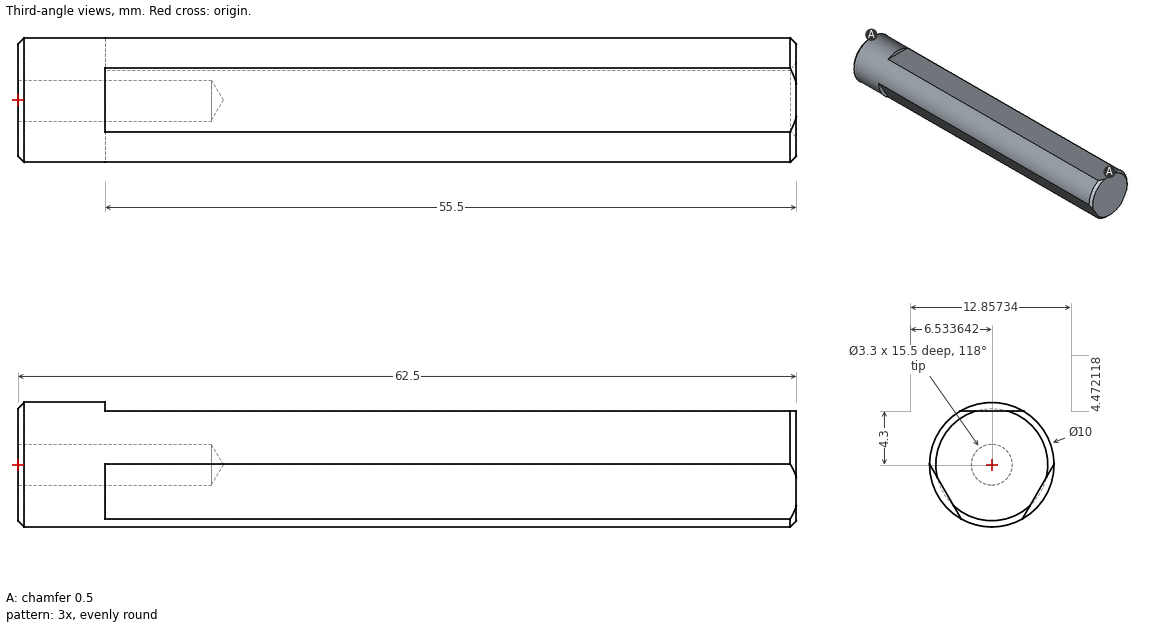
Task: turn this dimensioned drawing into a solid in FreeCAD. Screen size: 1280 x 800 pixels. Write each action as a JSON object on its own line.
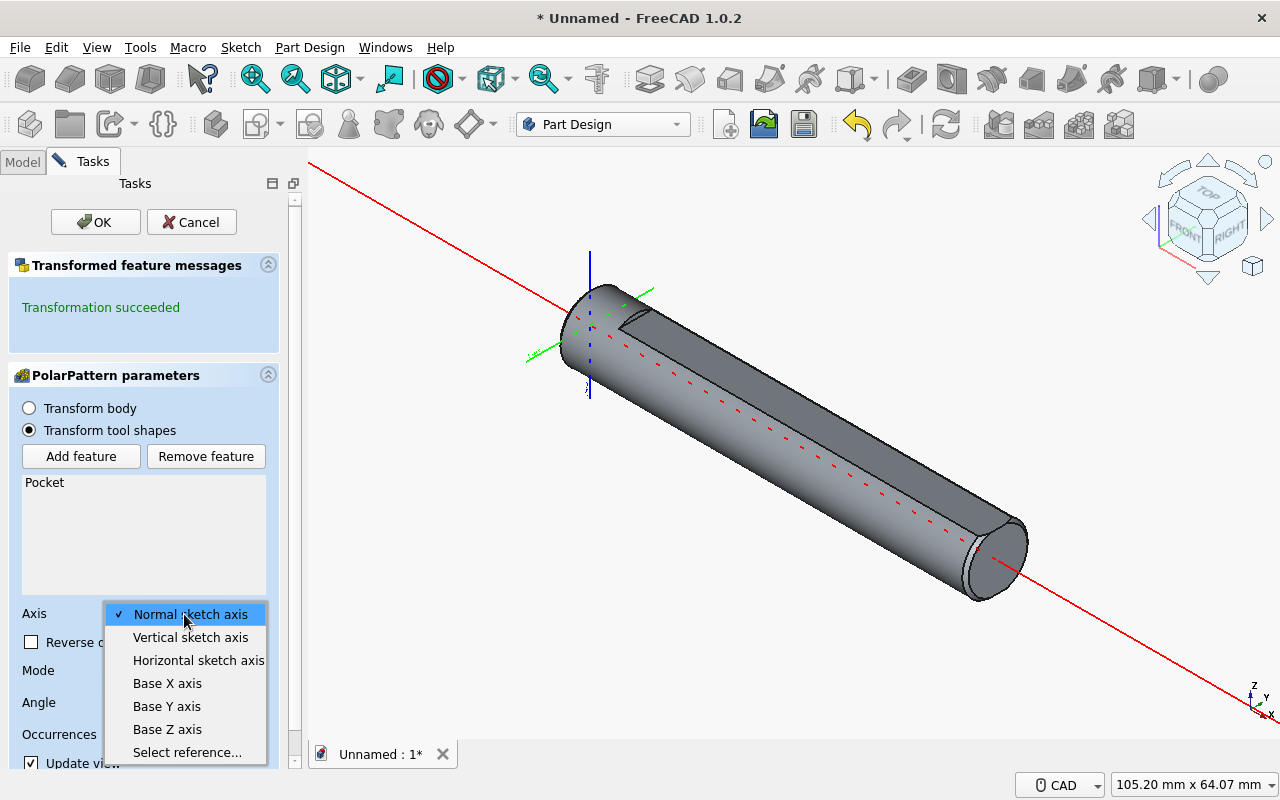
{"action": "left_click", "coordinate": [184, 684]}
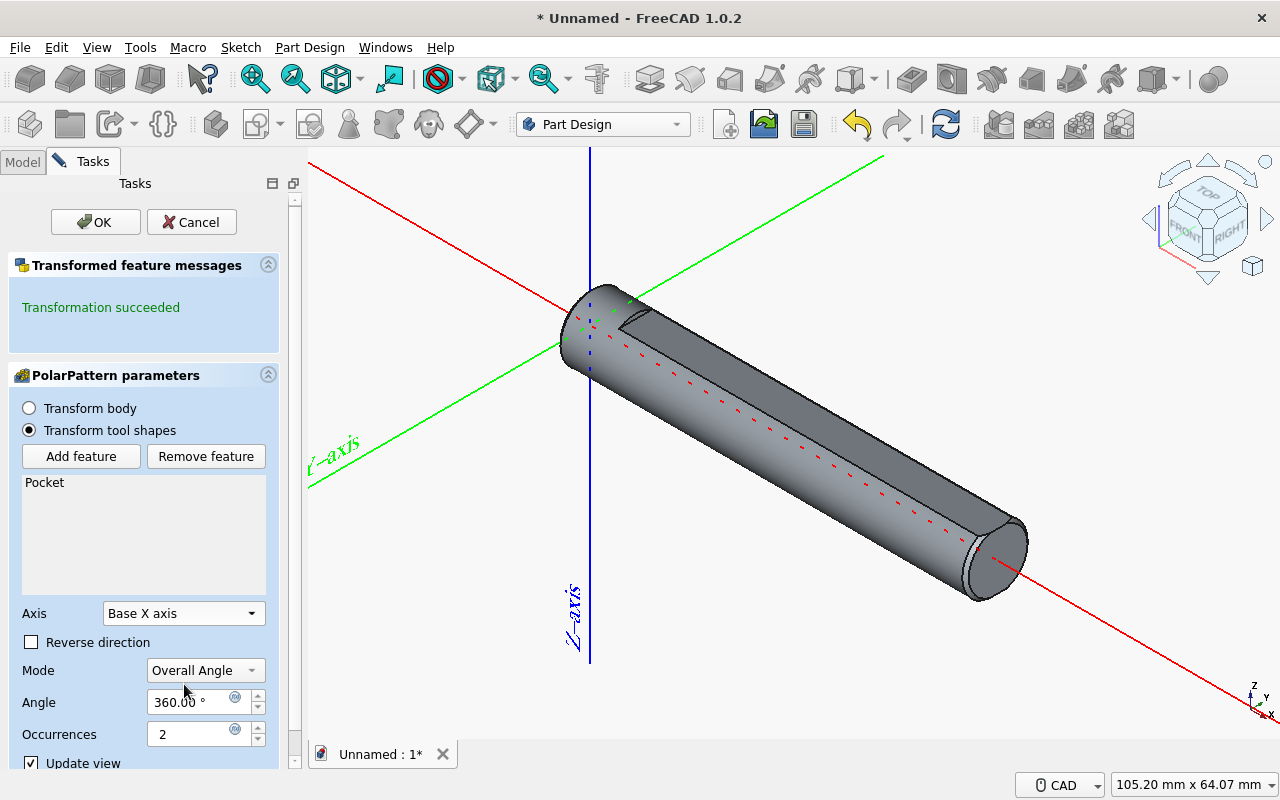
{"action": "triple_click", "coordinate": [198, 734]}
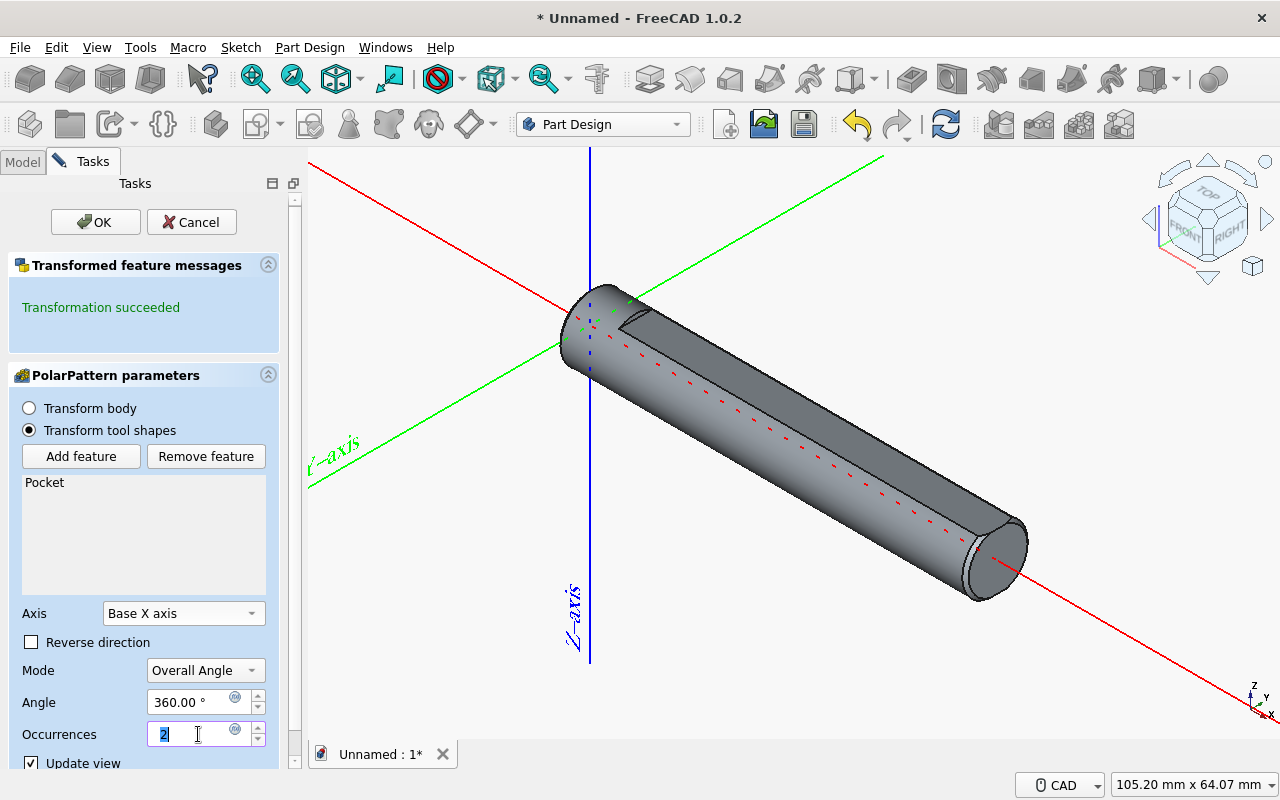
{"action": "type", "text": "3"}
{"action": "key", "text": "Tab"}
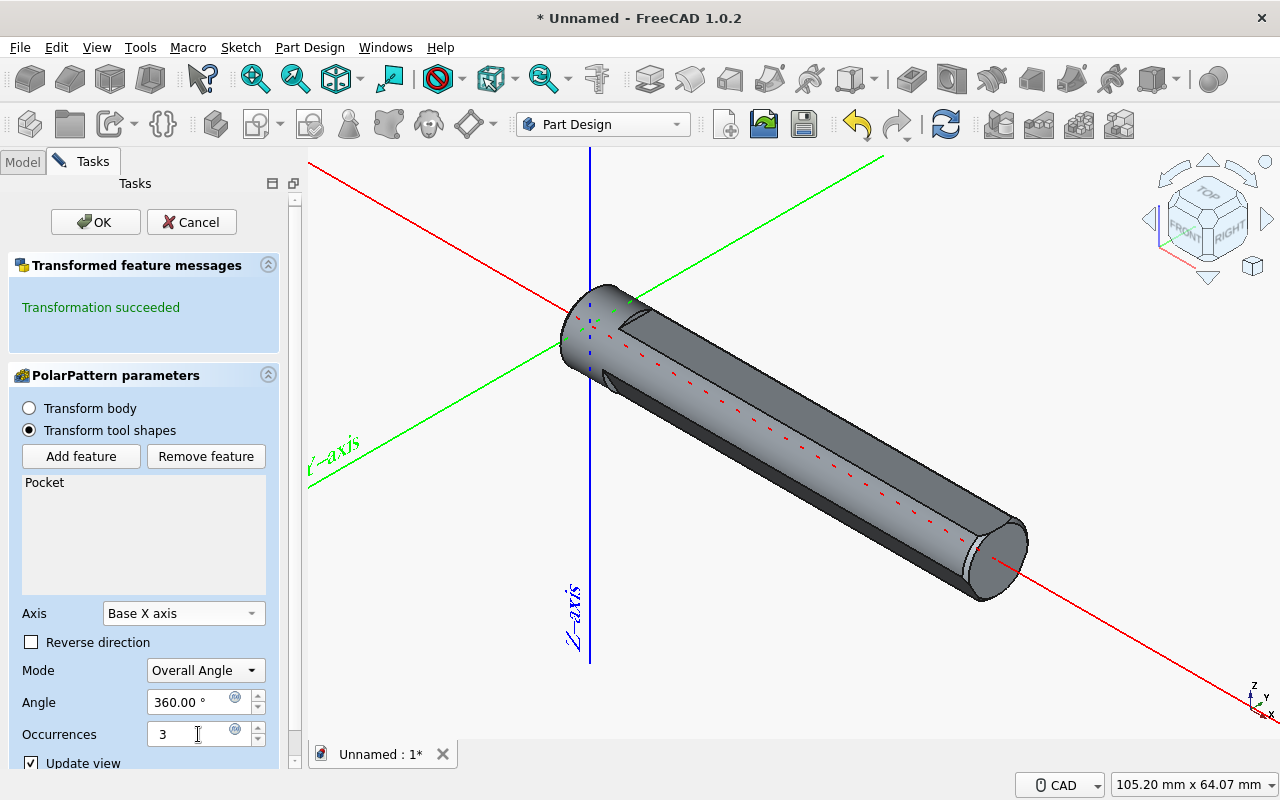
{"action": "left_click", "coordinate": [96, 222]}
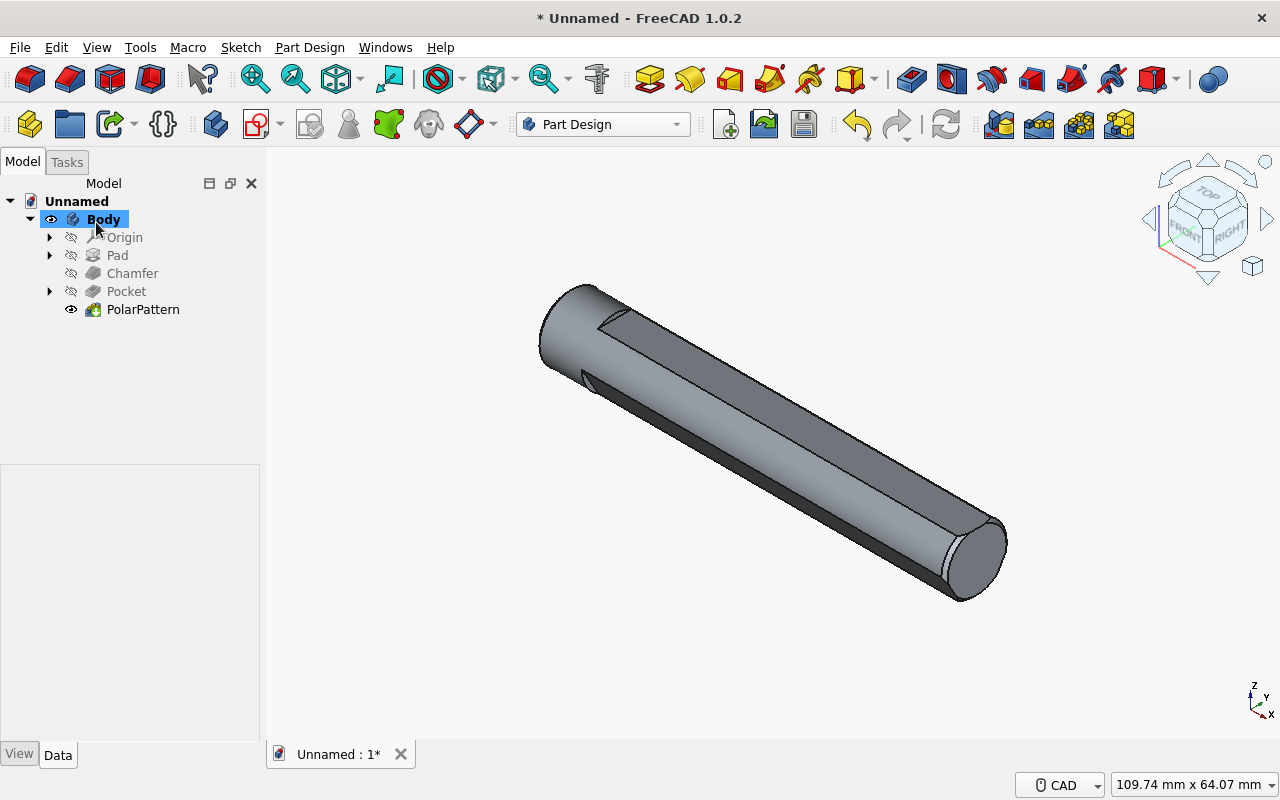
{"action": "key", "text": "6"}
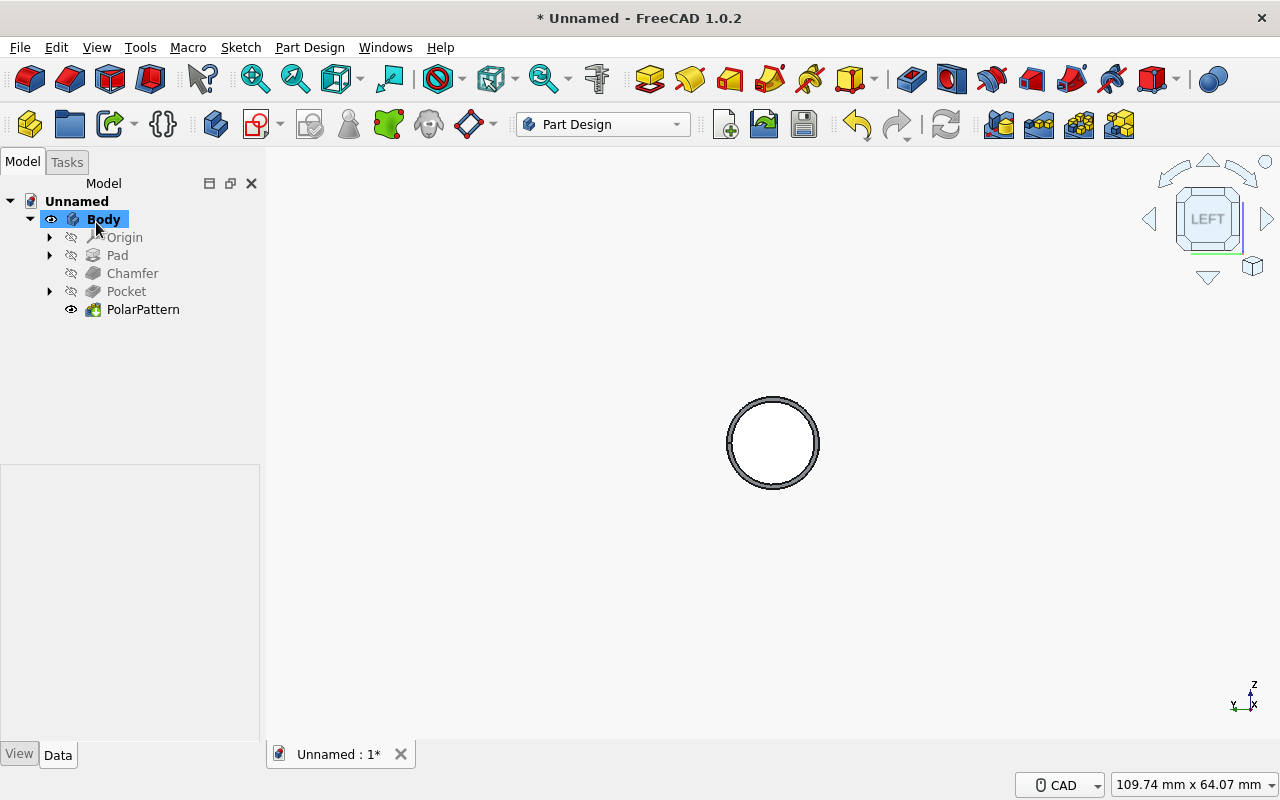
{"action": "left_click", "coordinate": [256, 80]}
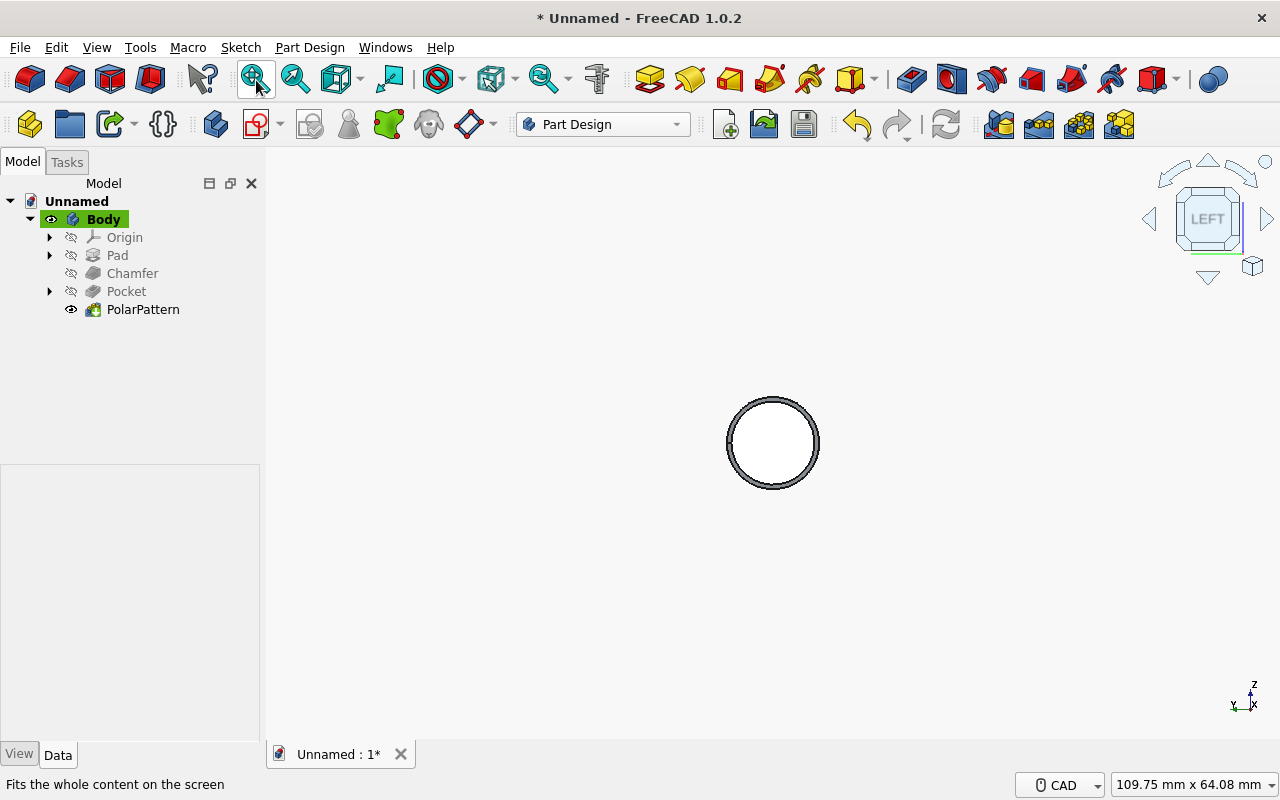
{"action": "left_click", "coordinate": [773, 442]}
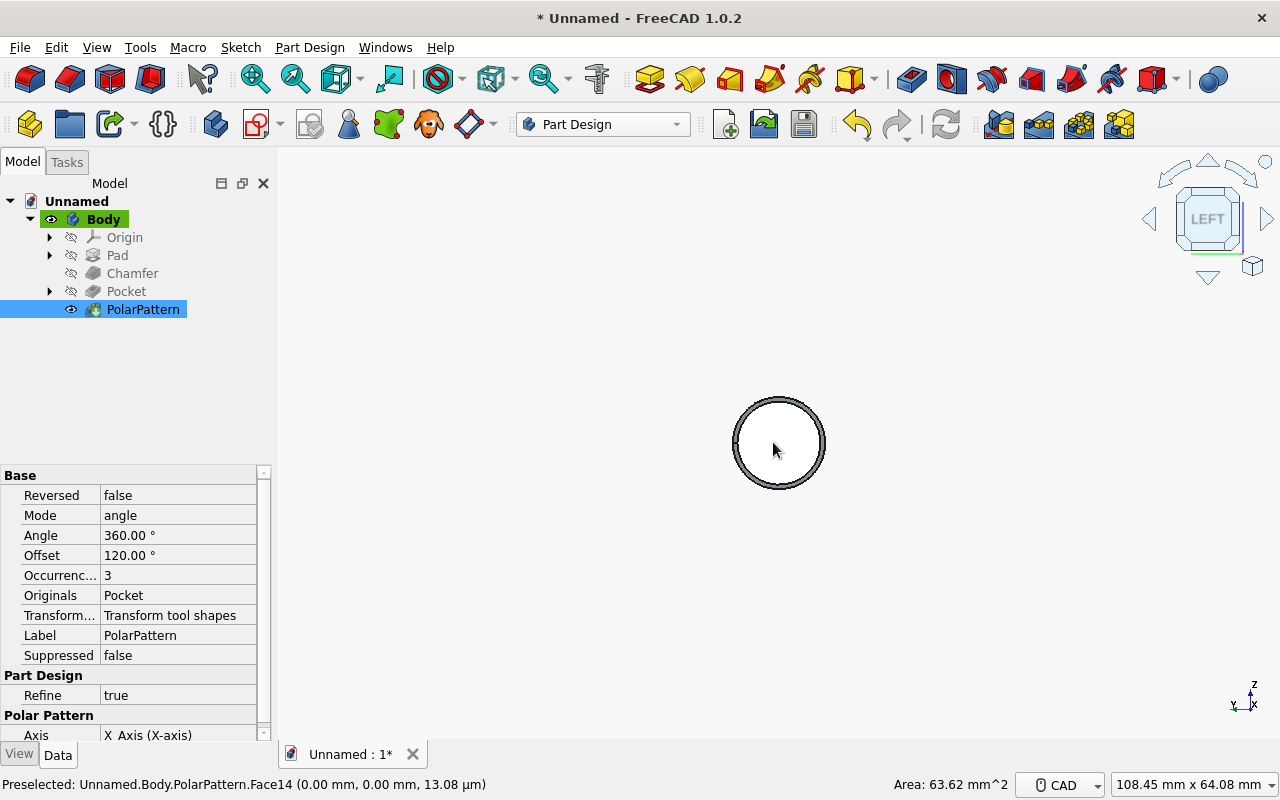
{"action": "left_click", "coordinate": [256, 124]}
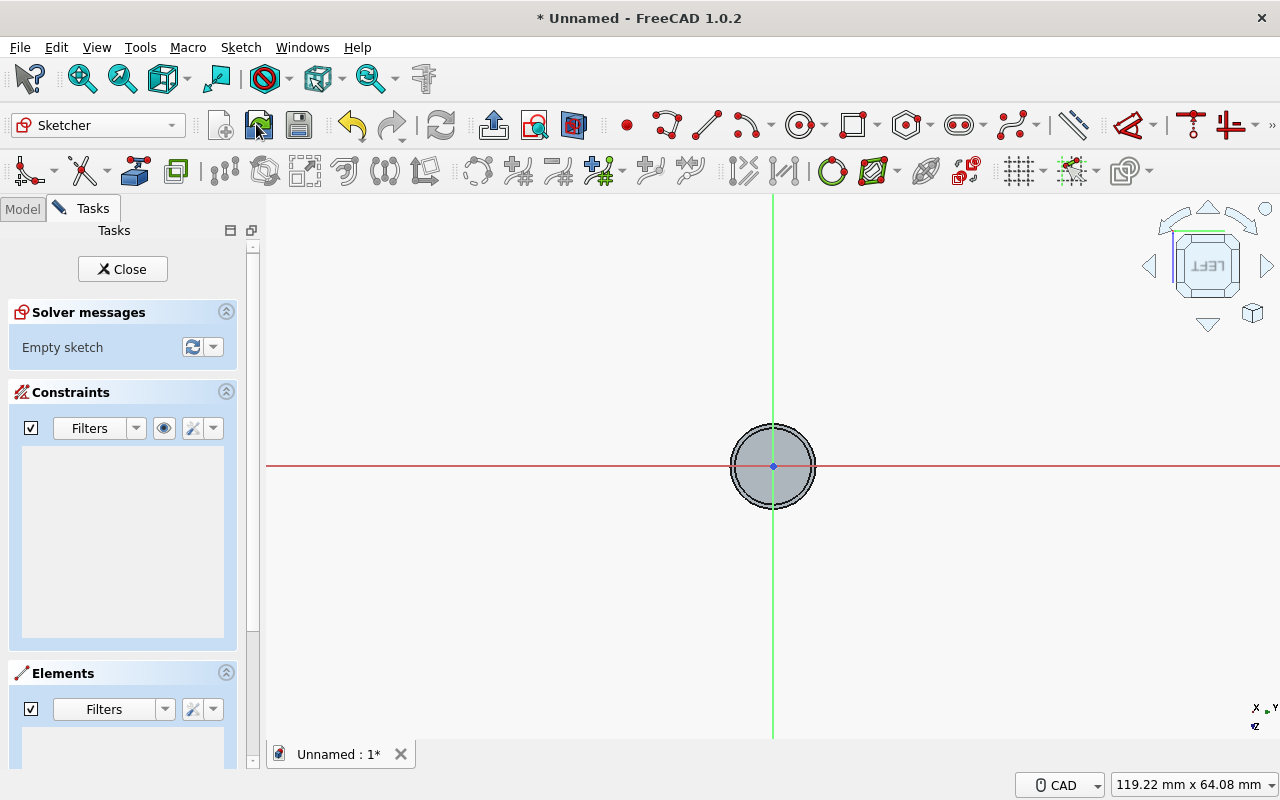
{"action": "scroll", "coordinate": [778, 466], "scroll_direction": "up", "scroll_amount": 13}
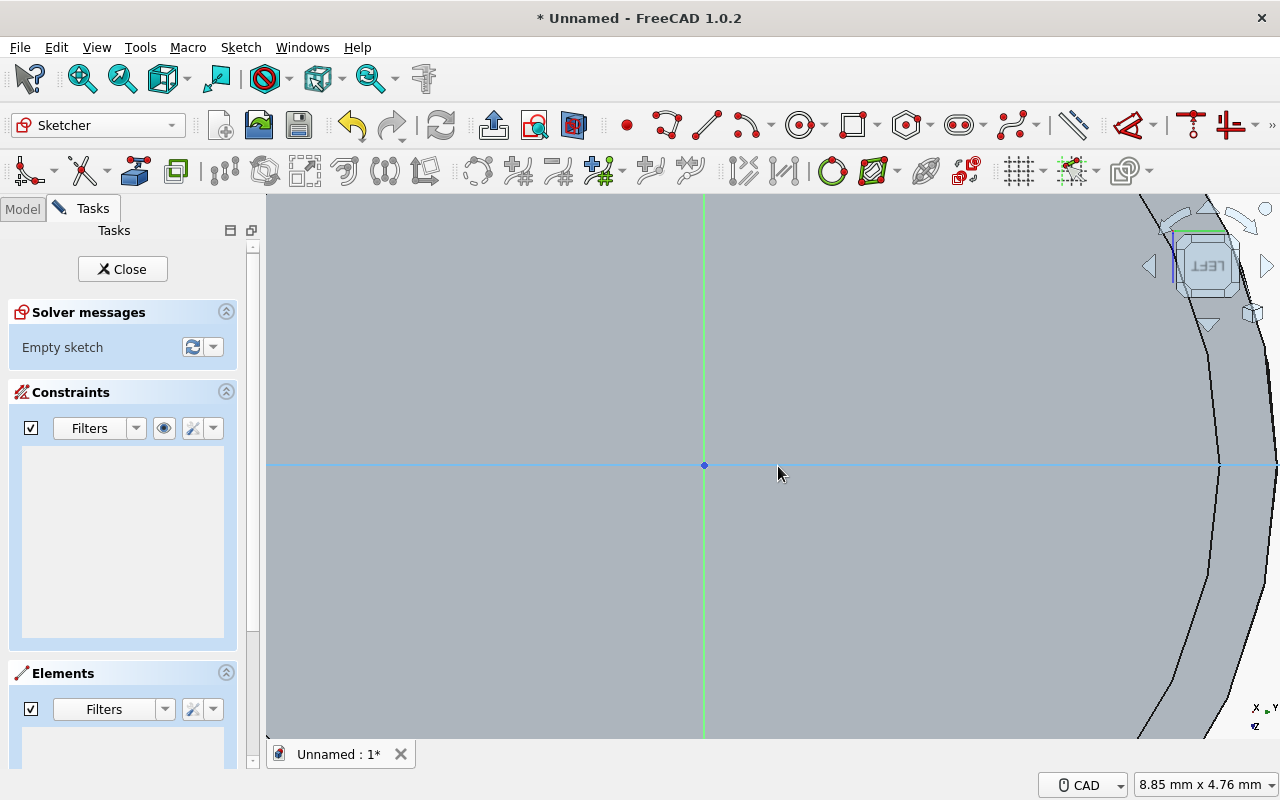
{"action": "left_click", "coordinate": [800, 126]}